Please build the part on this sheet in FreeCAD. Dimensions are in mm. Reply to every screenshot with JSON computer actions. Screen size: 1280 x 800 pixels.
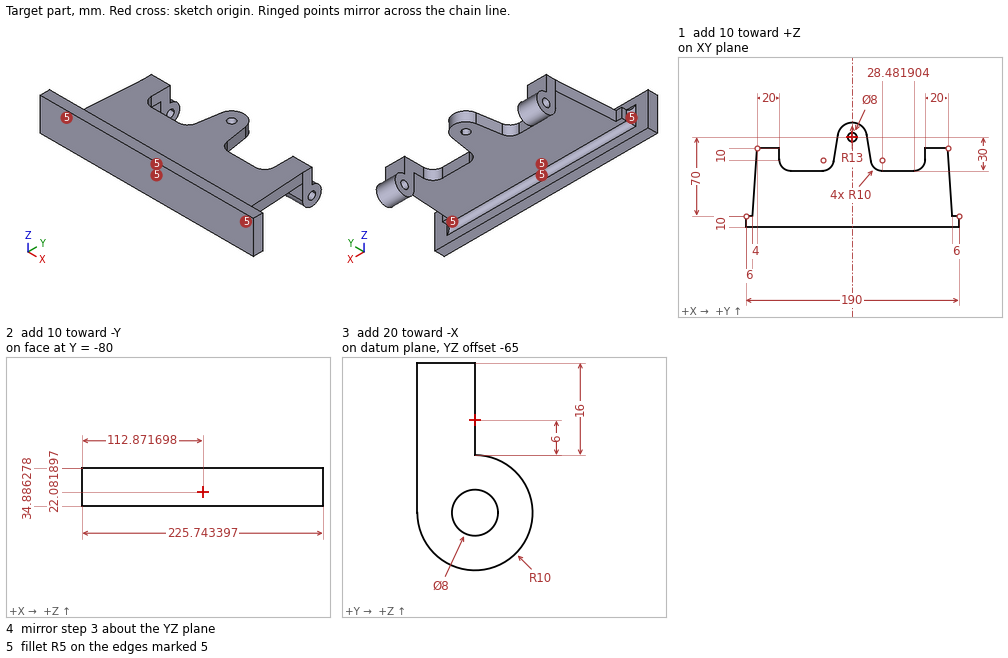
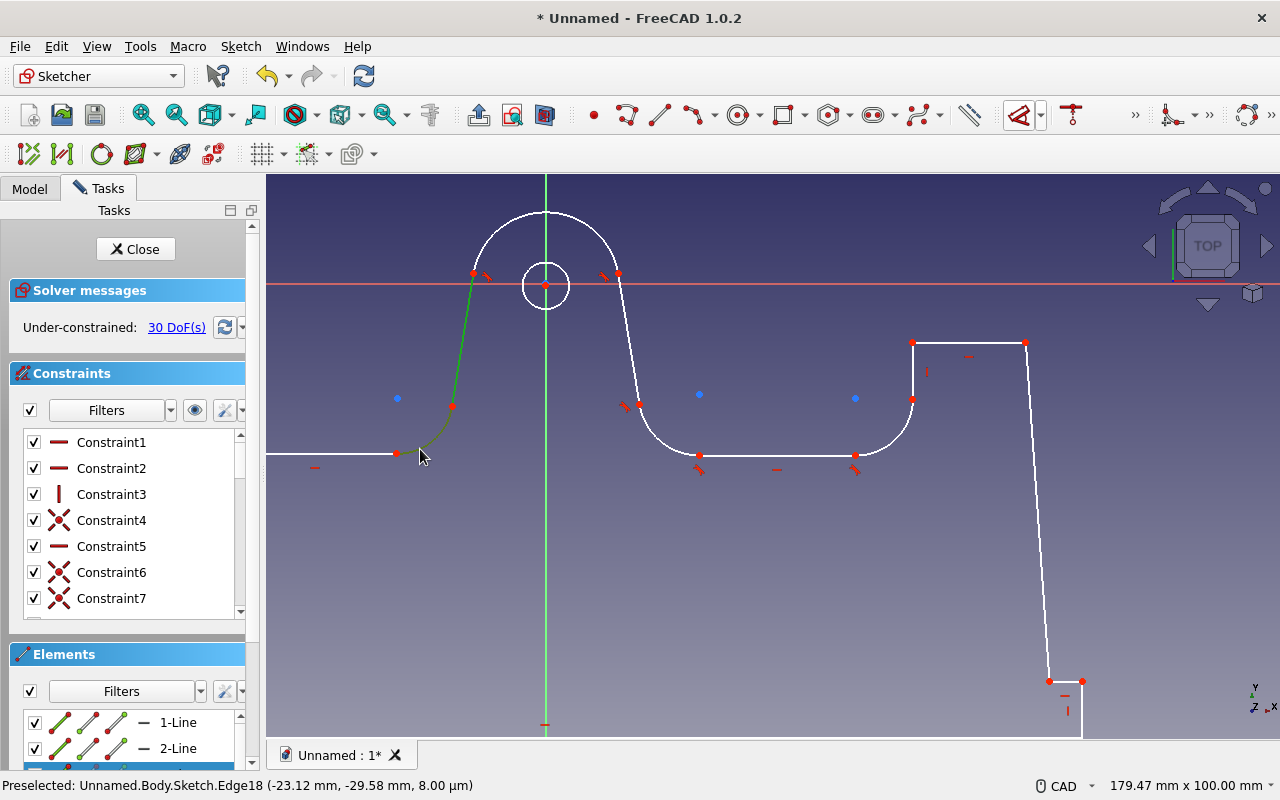
{"action": "key", "text": "t"}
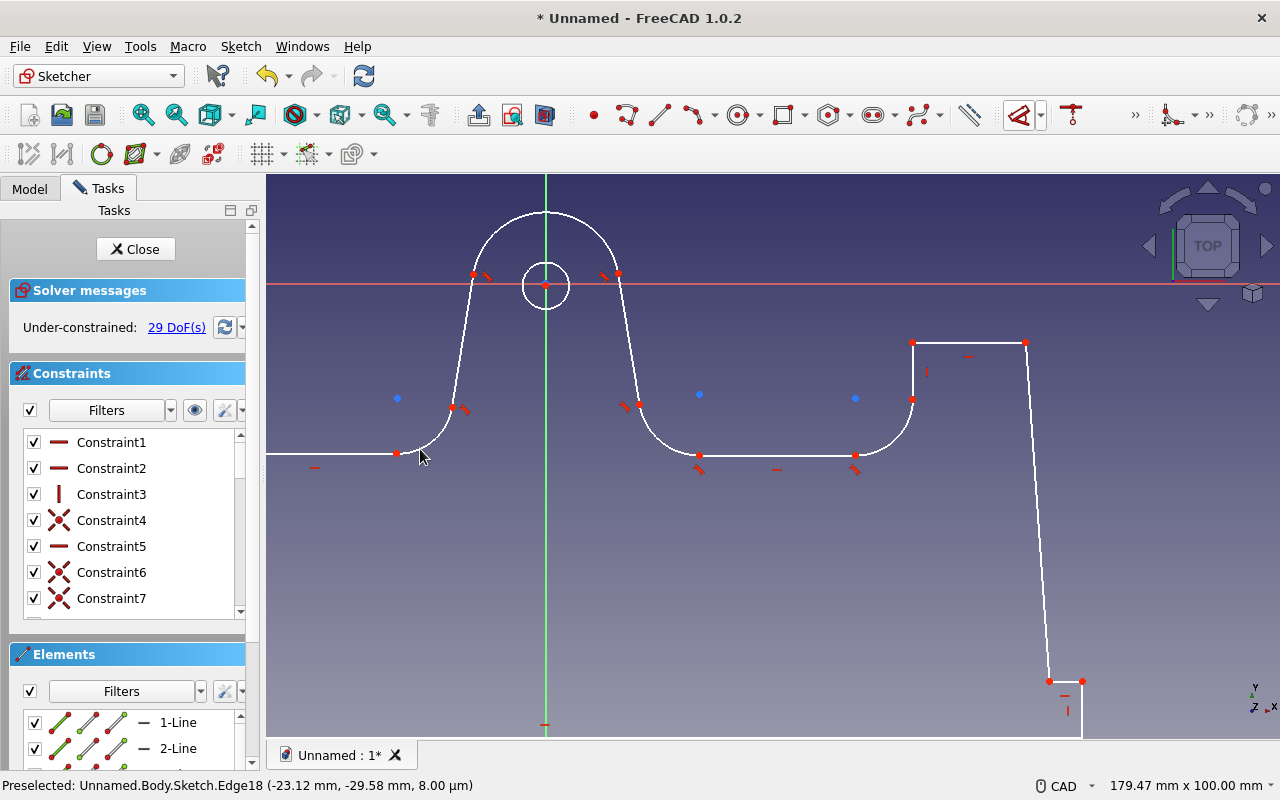
{"action": "left_click", "coordinate": [348, 454]}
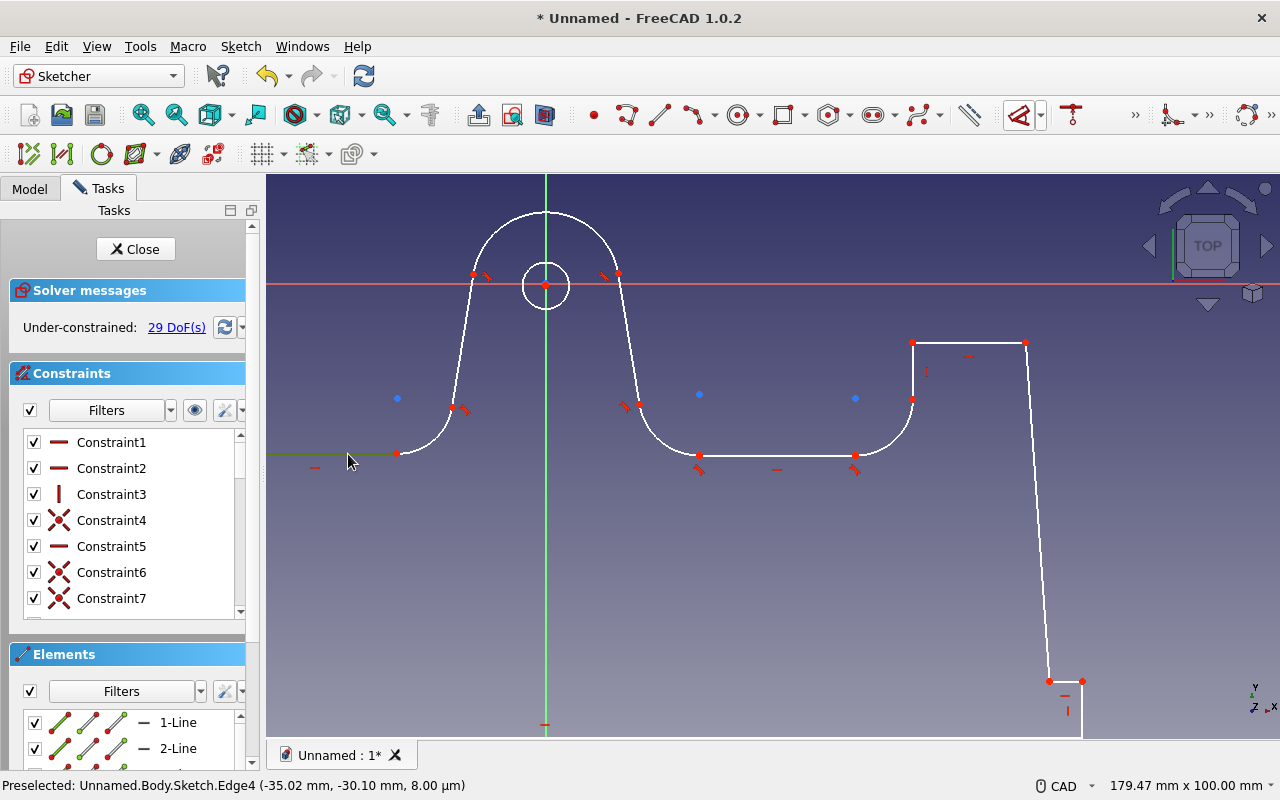
{"action": "left_click", "coordinate": [419, 449]}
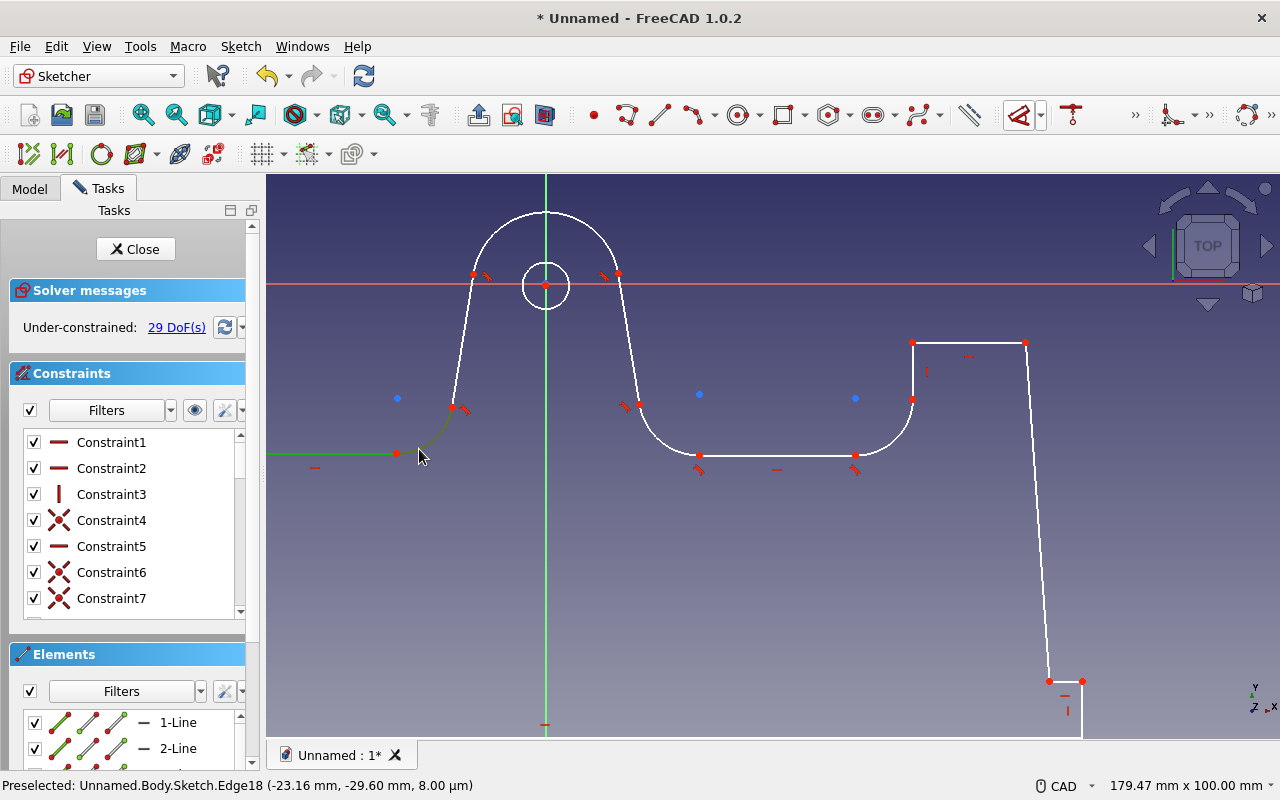
{"action": "key", "text": "t"}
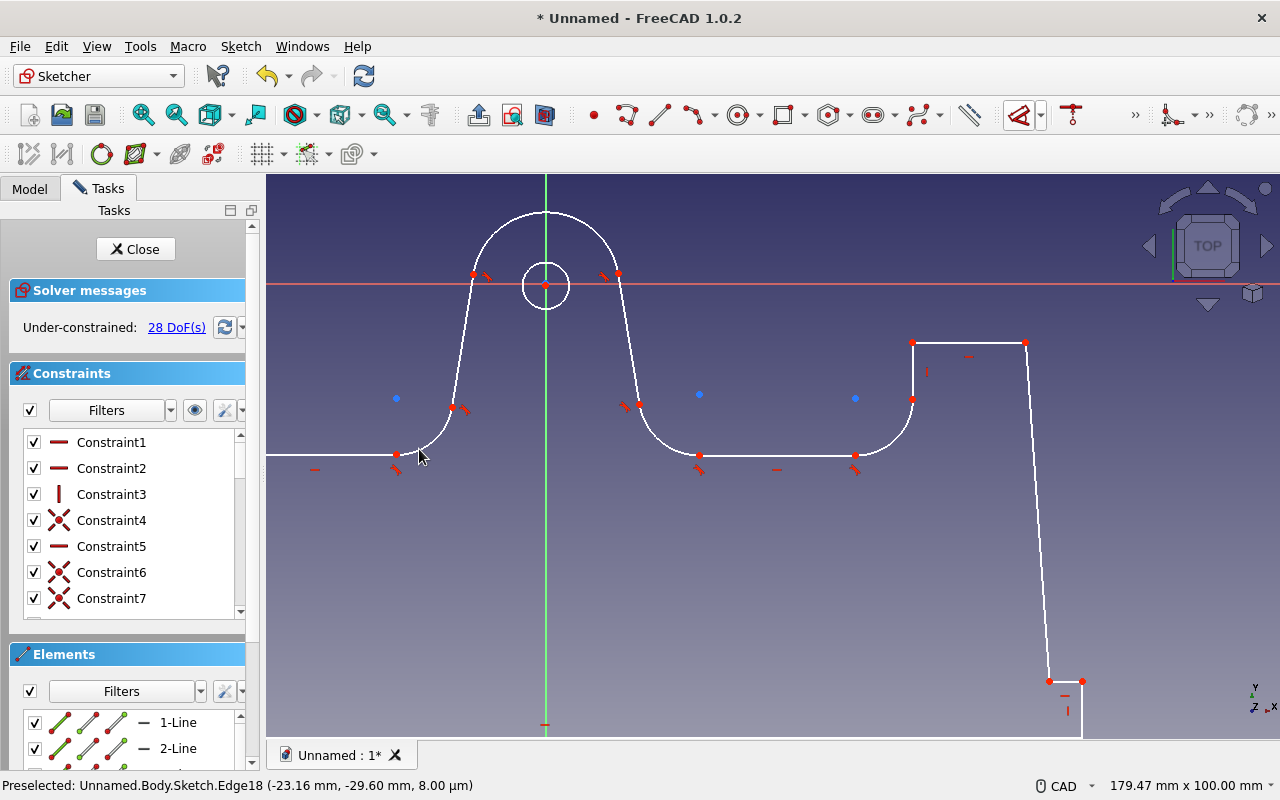
{"action": "left_click", "coordinate": [348, 455]}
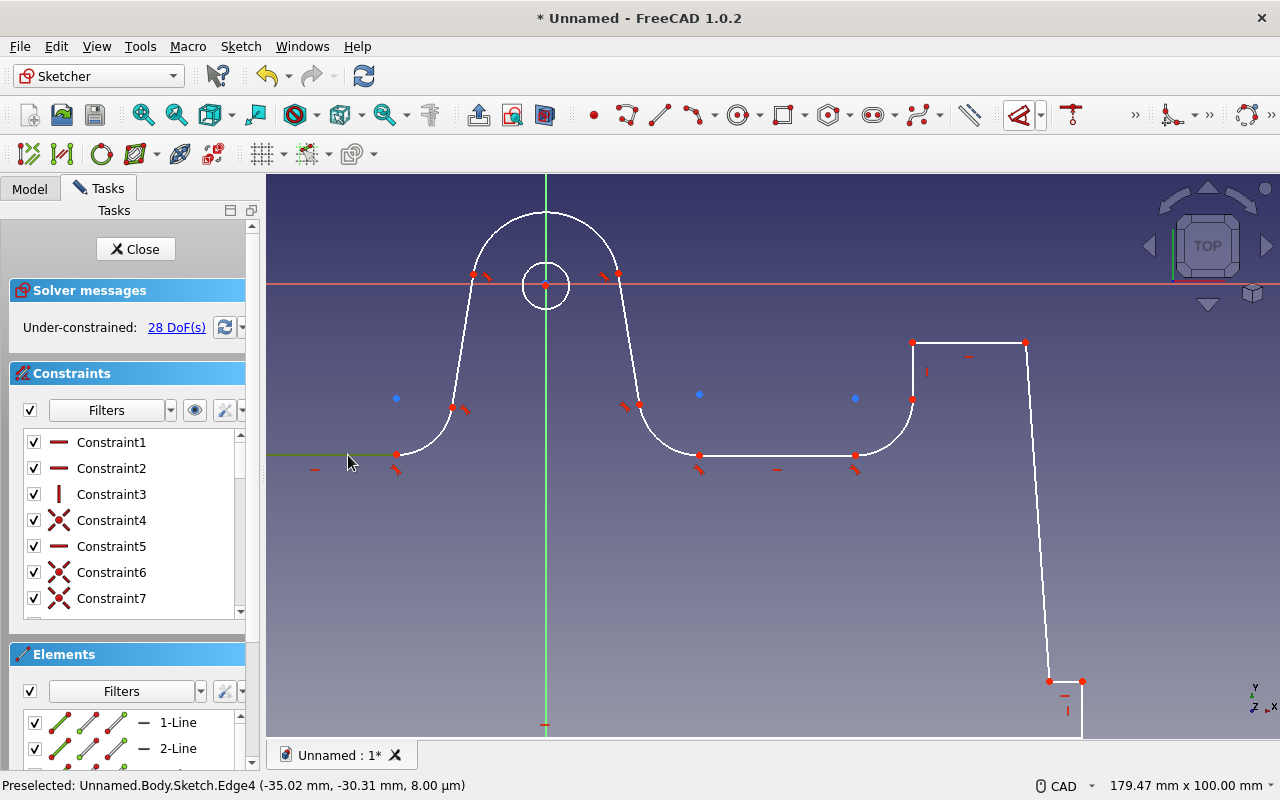
{"action": "scroll", "coordinate": [897, 436], "scroll_direction": "down", "scroll_amount": 3}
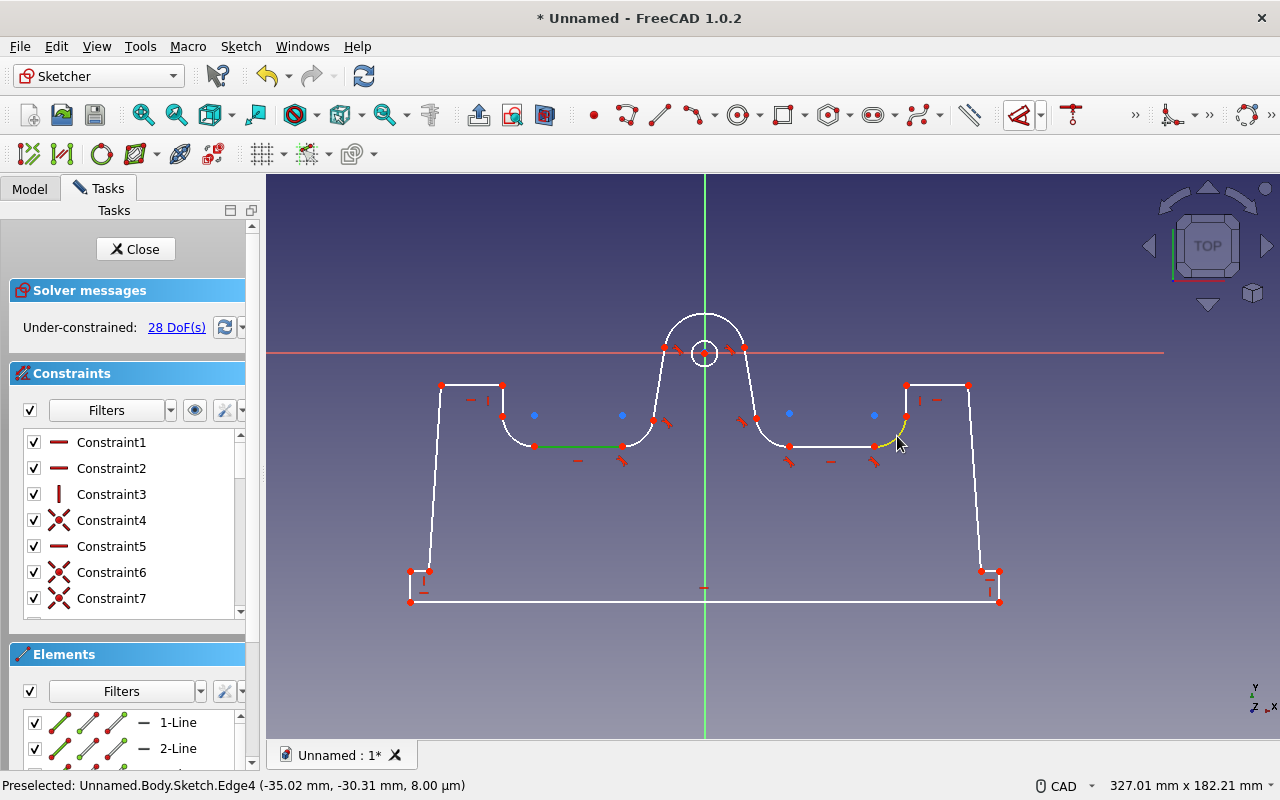
{"action": "left_click", "coordinate": [506, 430]}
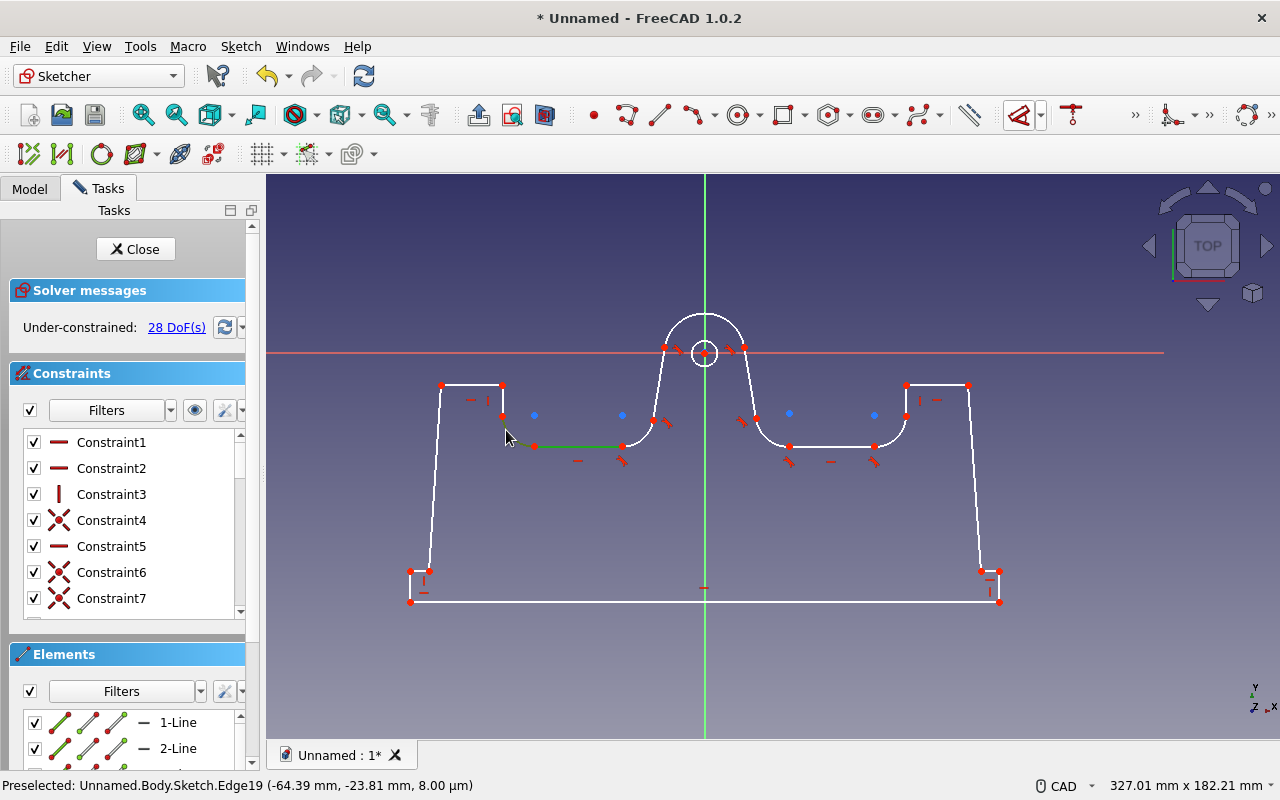
{"action": "key", "text": "t"}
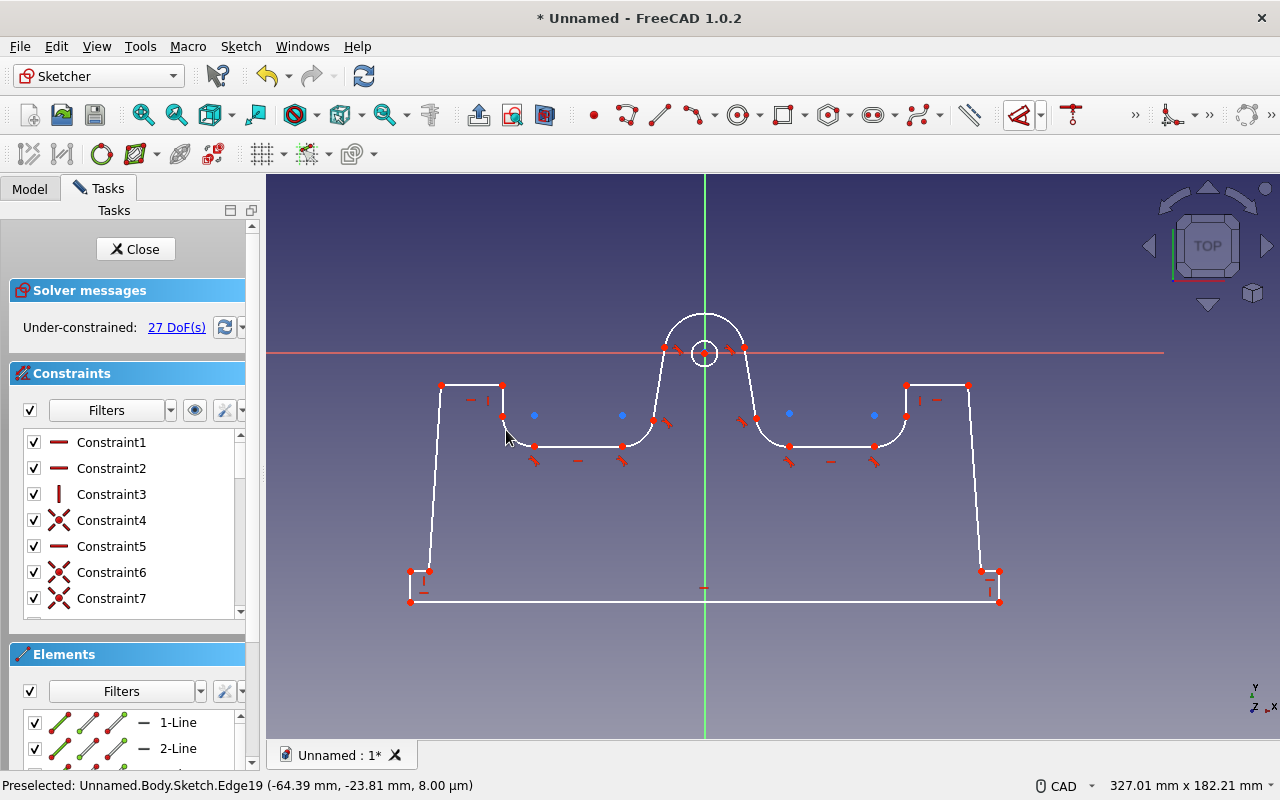
{"action": "scroll", "coordinate": [503, 407], "scroll_direction": "up", "scroll_amount": 2}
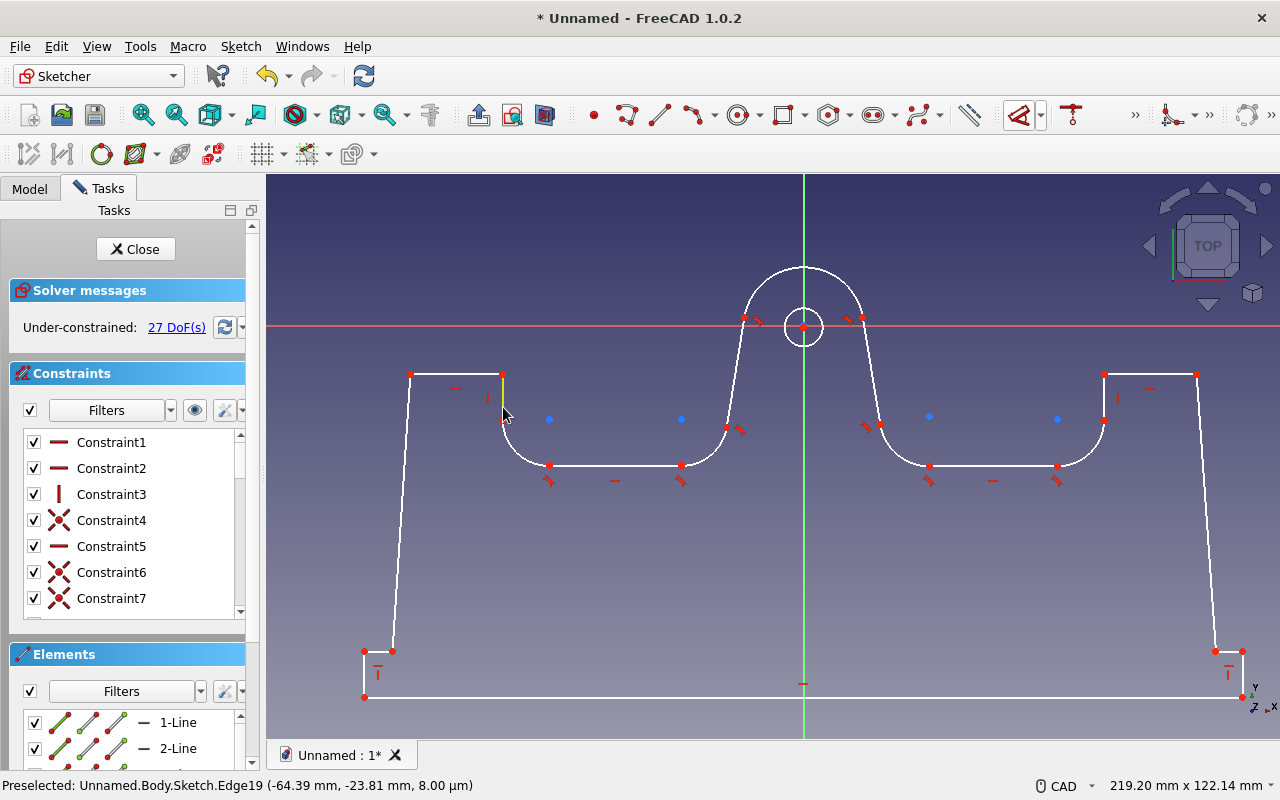
{"action": "left_click", "coordinate": [503, 406]}